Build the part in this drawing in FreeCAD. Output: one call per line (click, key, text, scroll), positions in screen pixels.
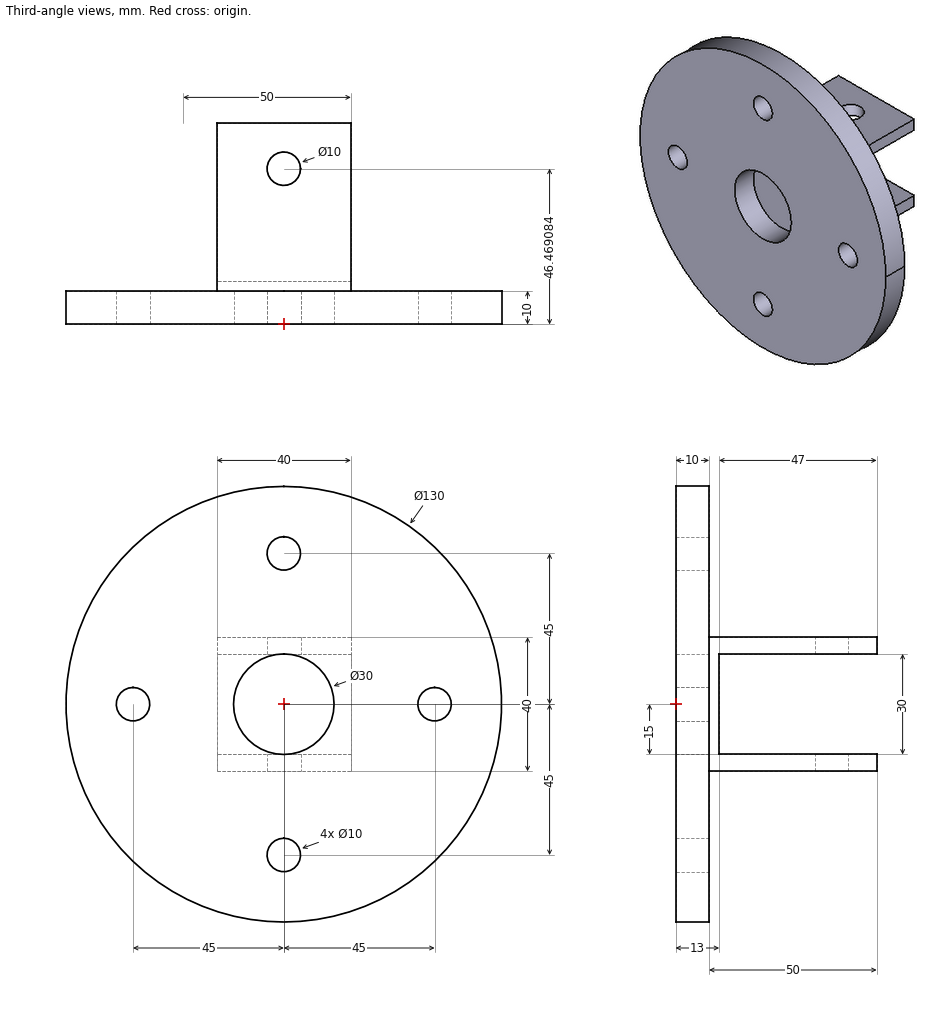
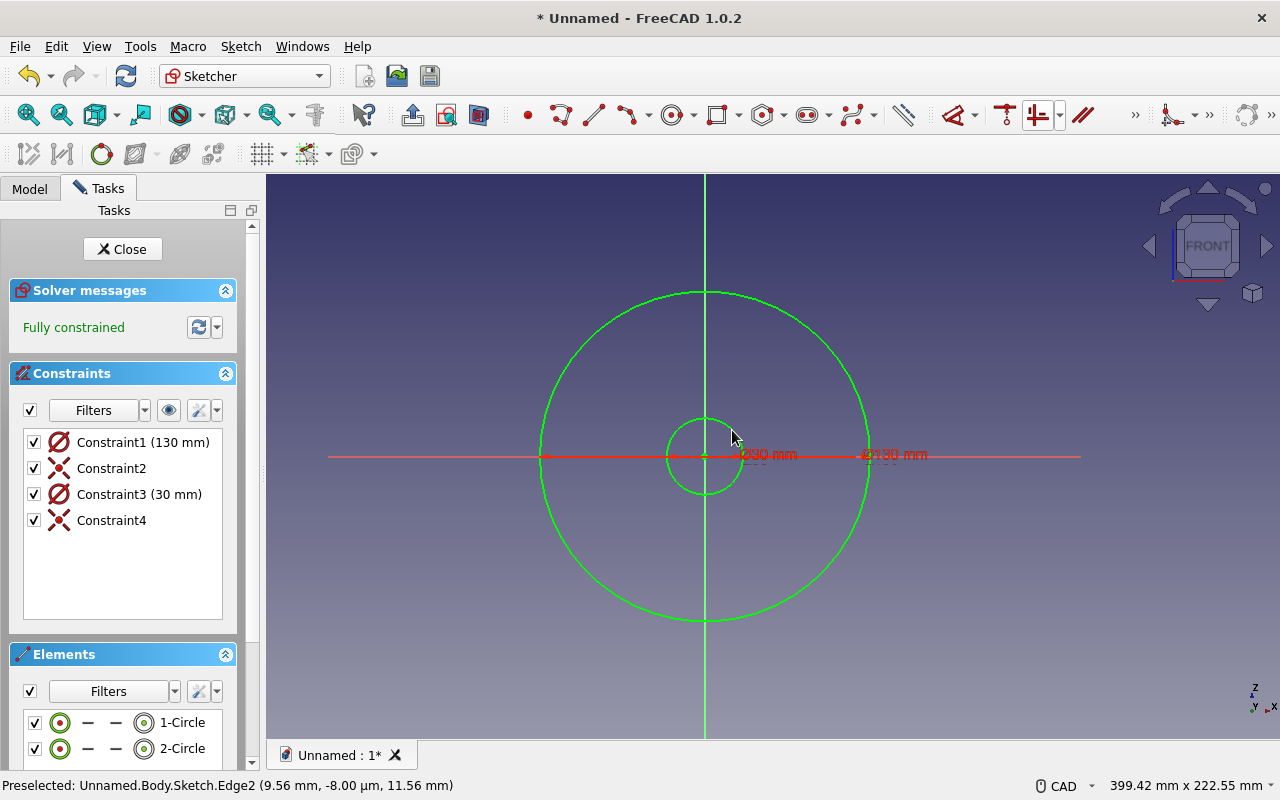
click(123, 249)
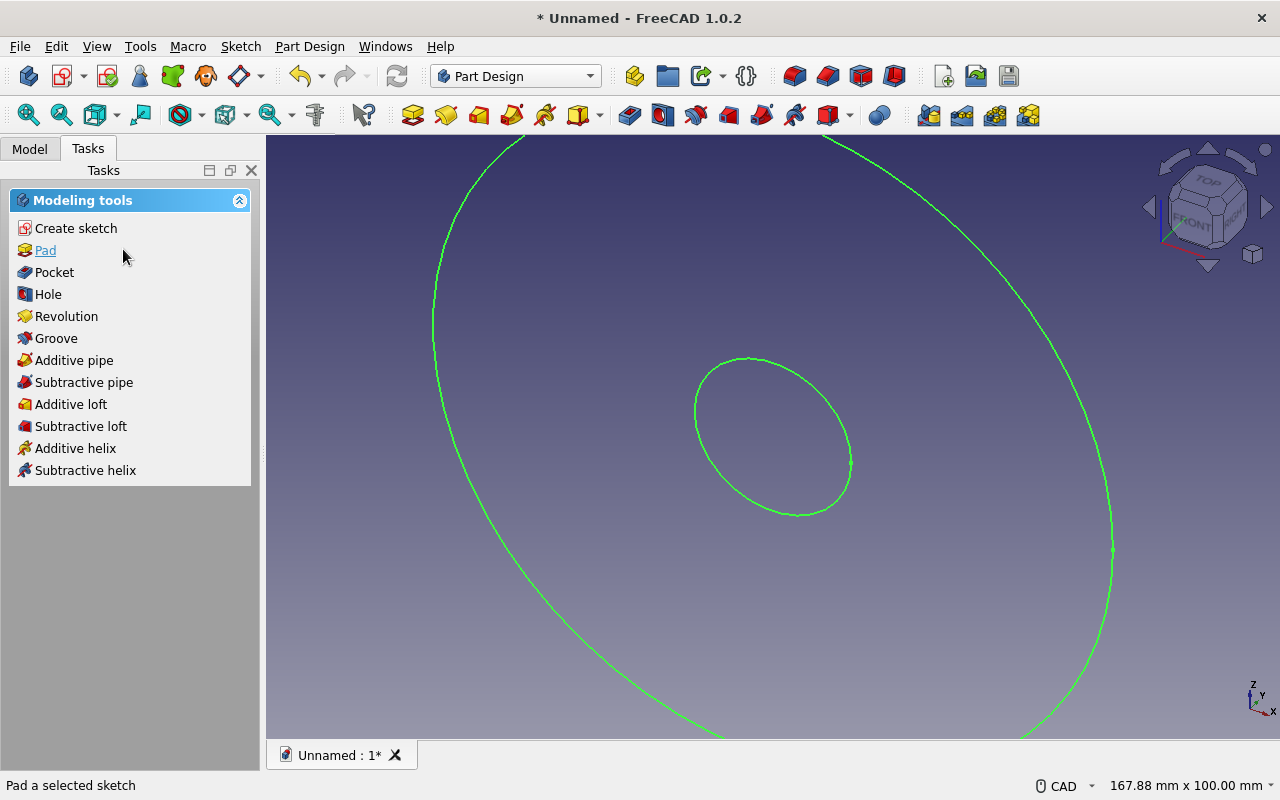
click(413, 116)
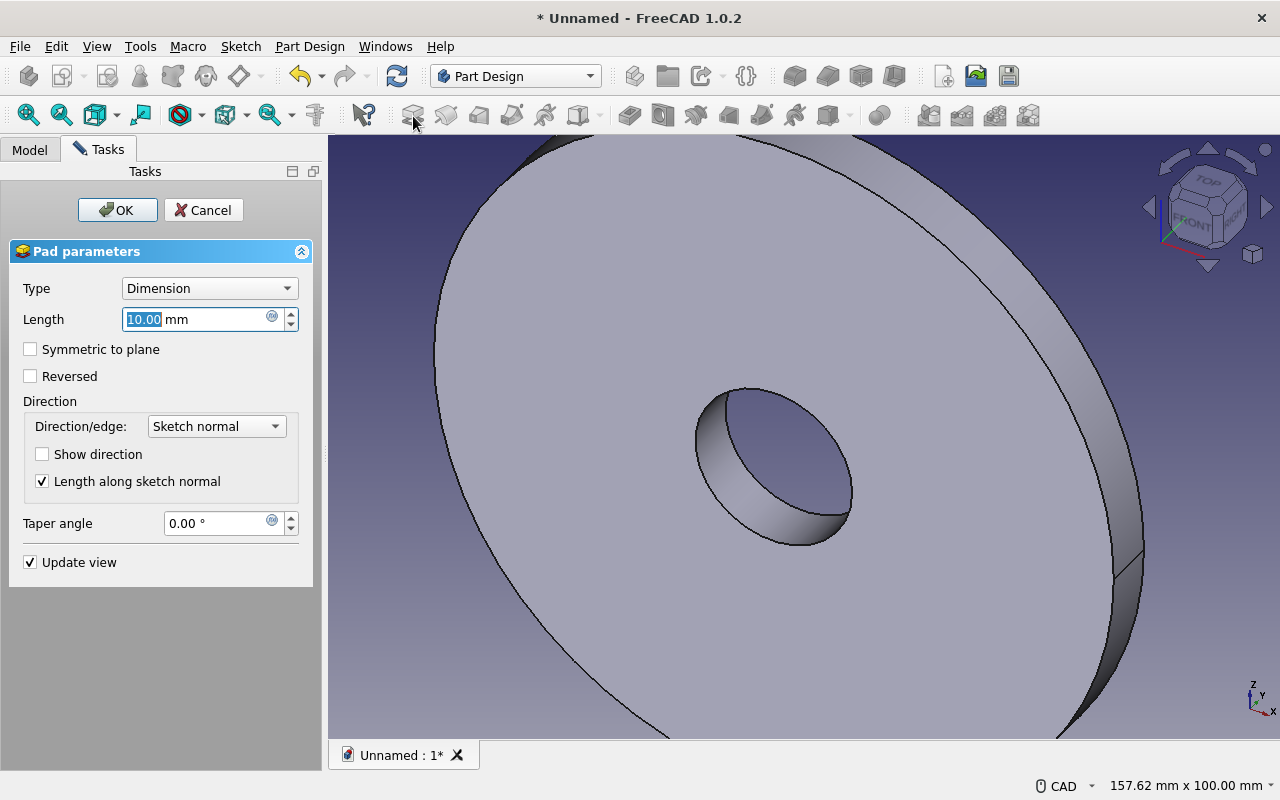
text(10)
key(Tab)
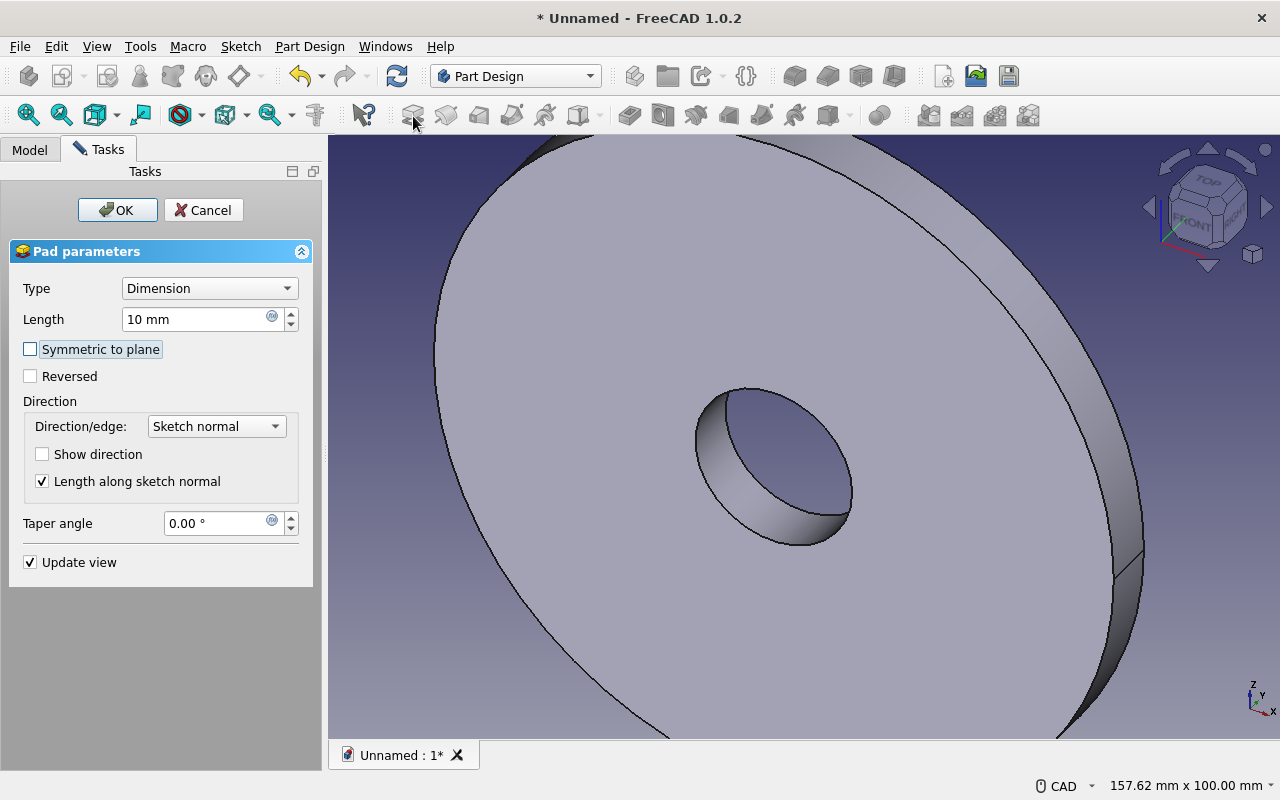
click(31, 376)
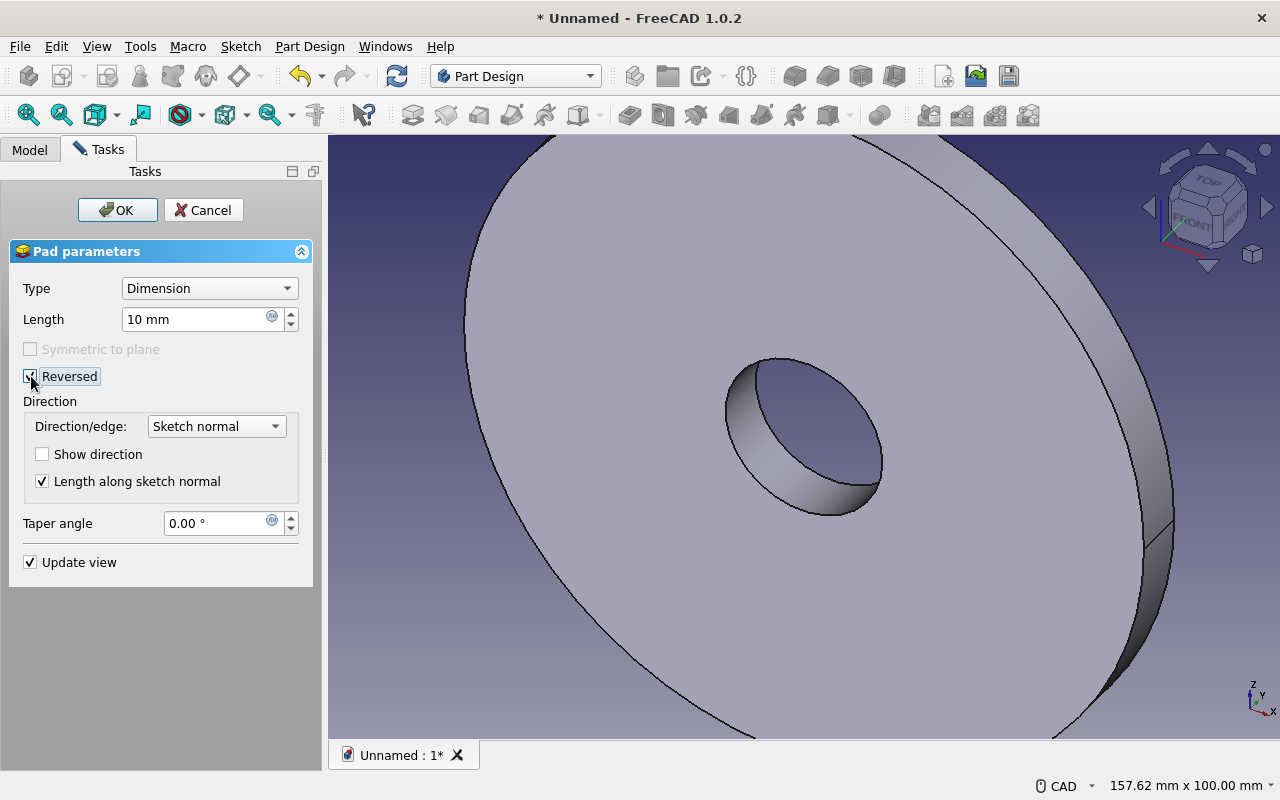
click(118, 210)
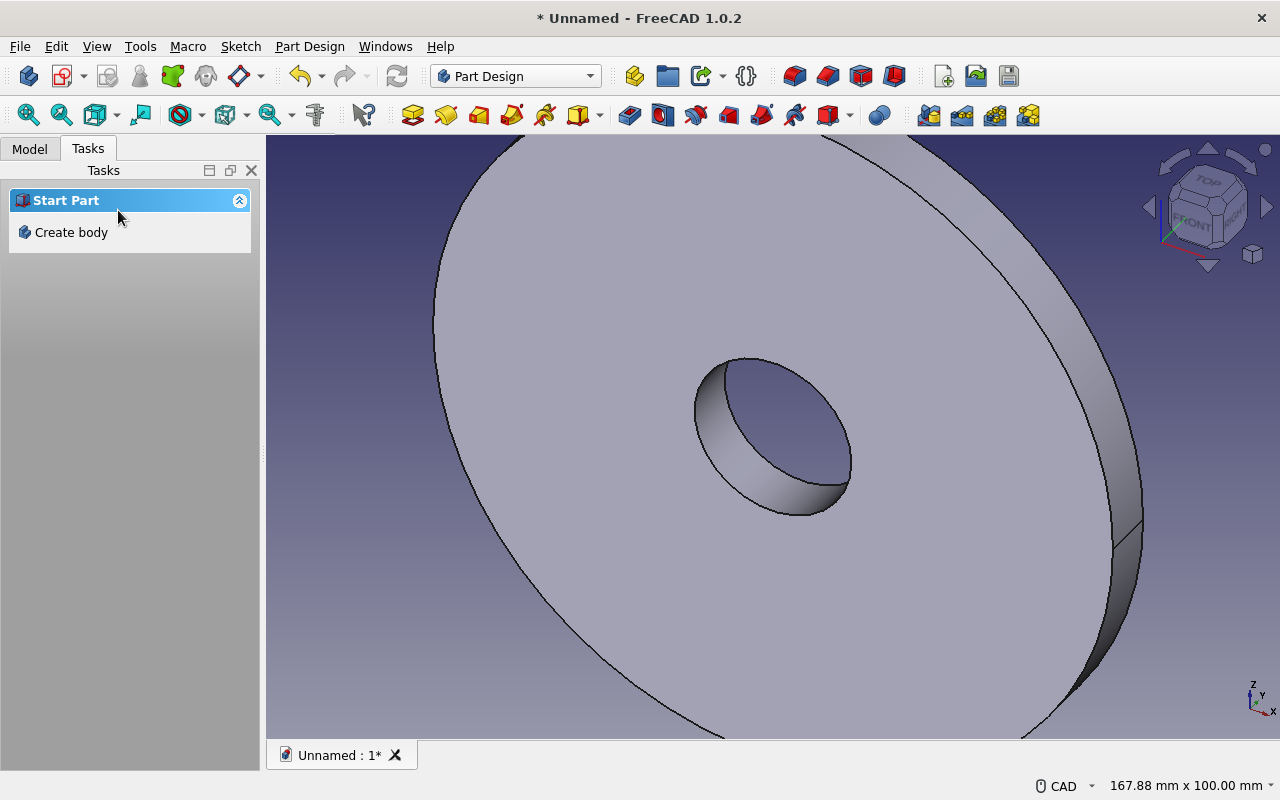
key(v)
key(f)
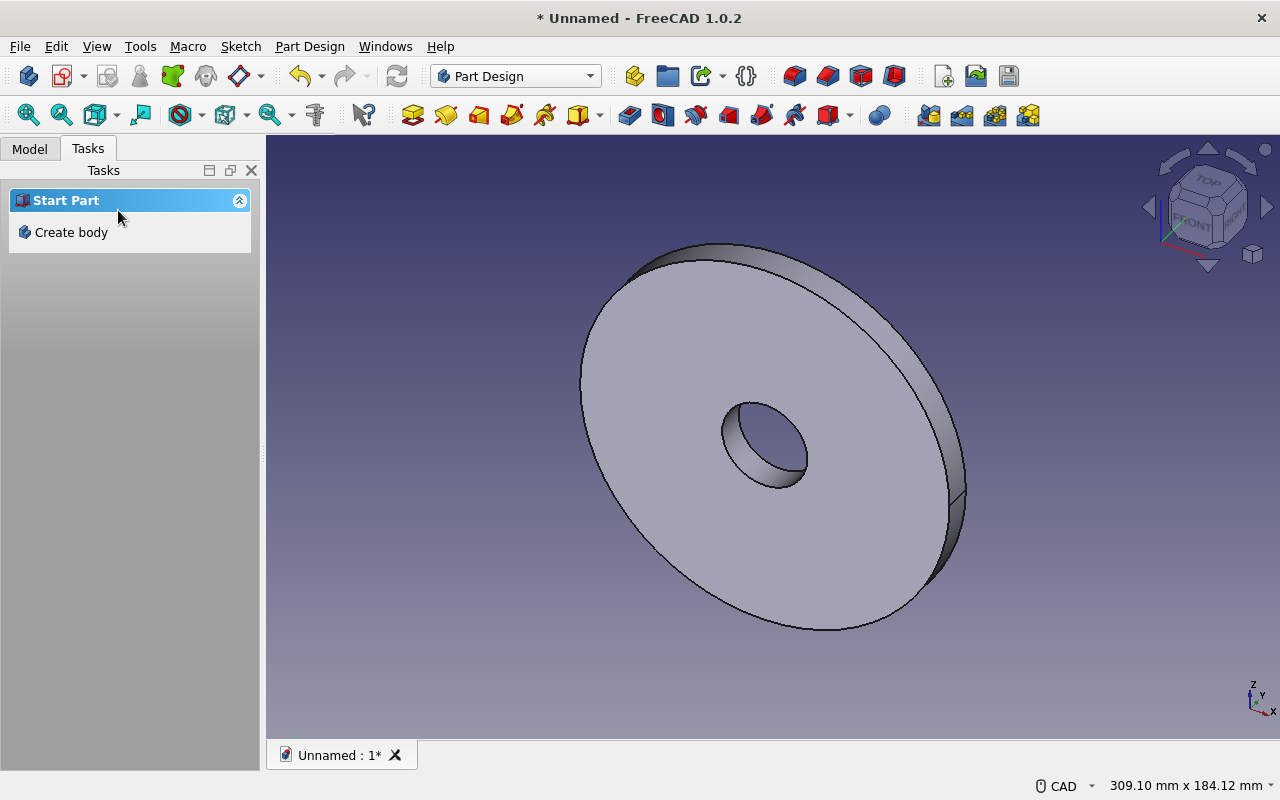
key(4)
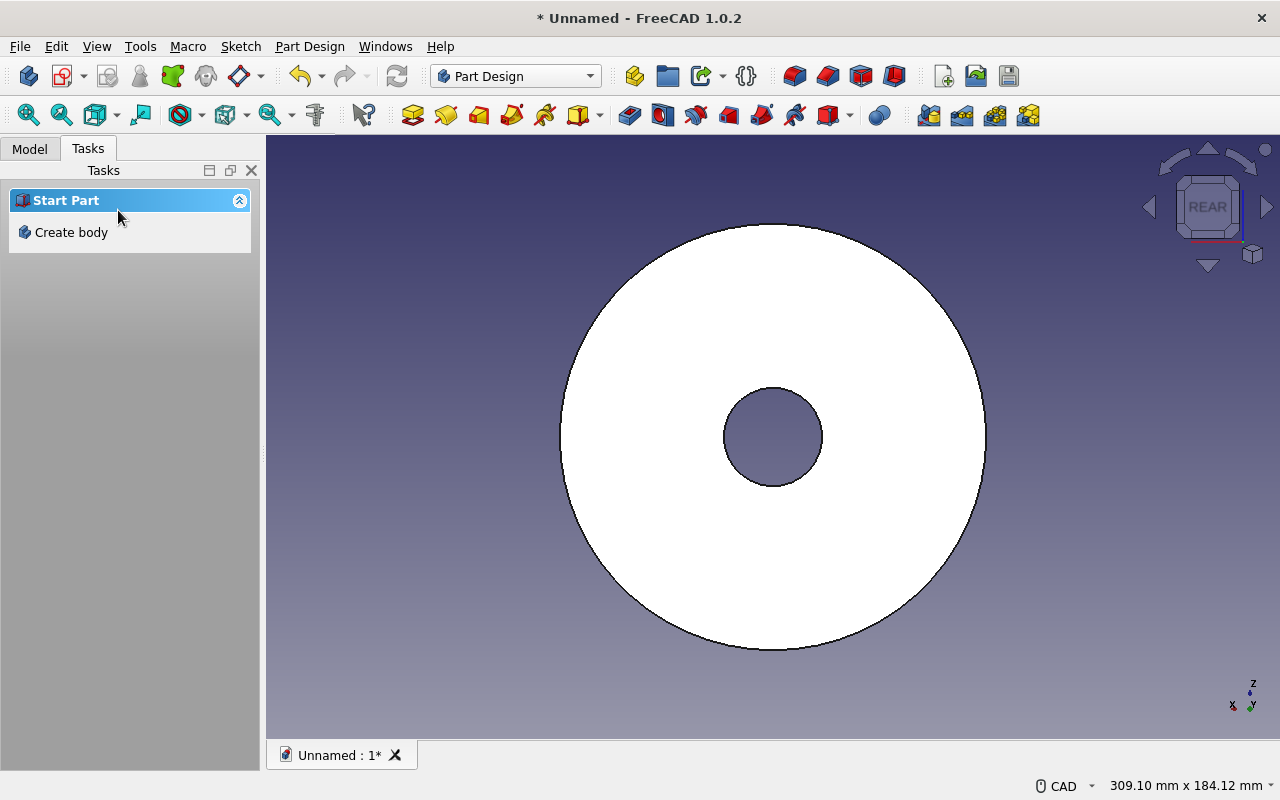
click(651, 497)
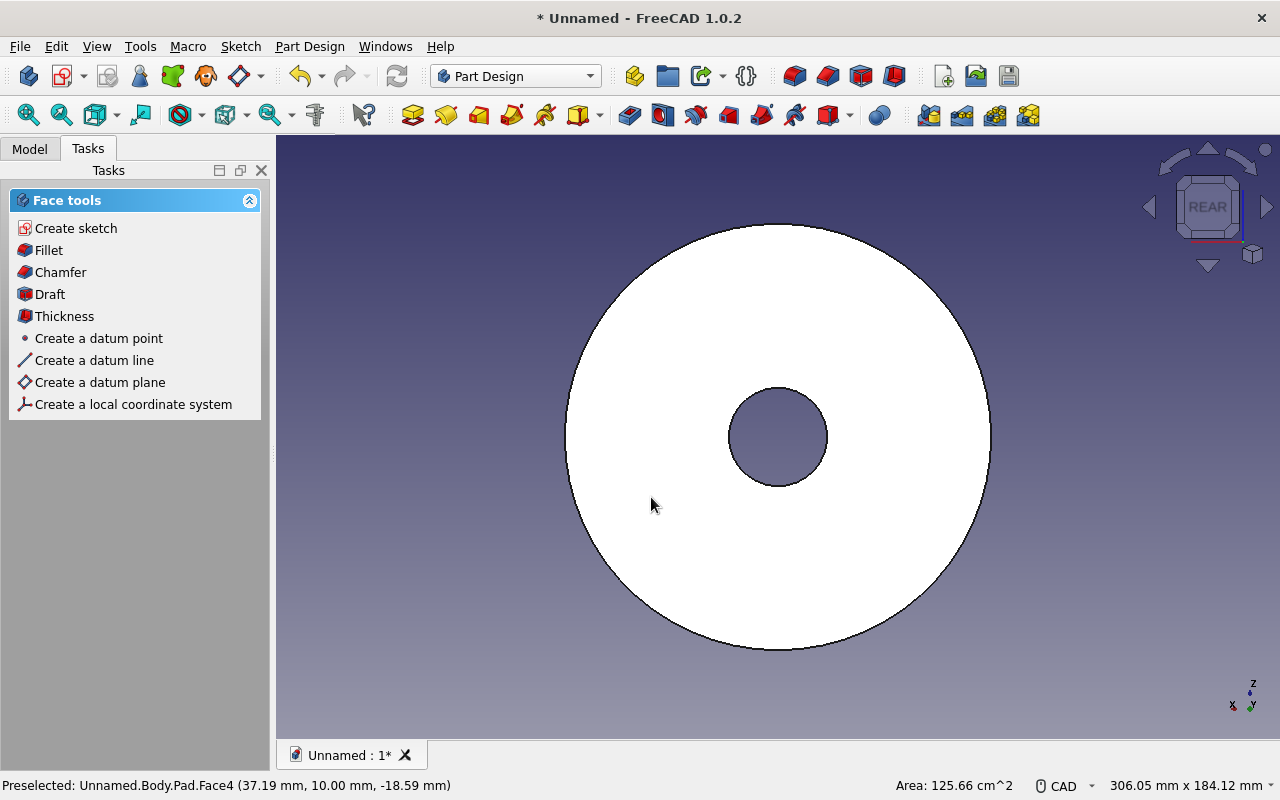
click(62, 76)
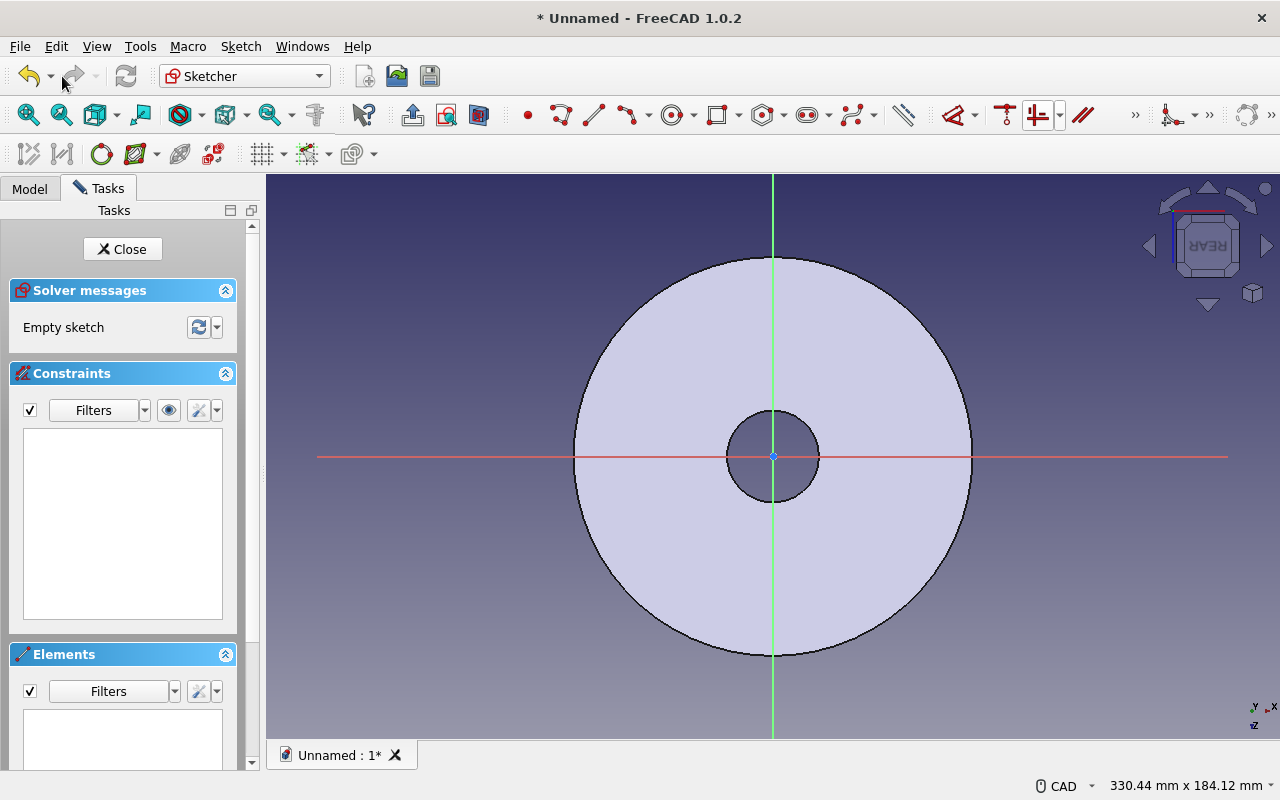
click(672, 116)